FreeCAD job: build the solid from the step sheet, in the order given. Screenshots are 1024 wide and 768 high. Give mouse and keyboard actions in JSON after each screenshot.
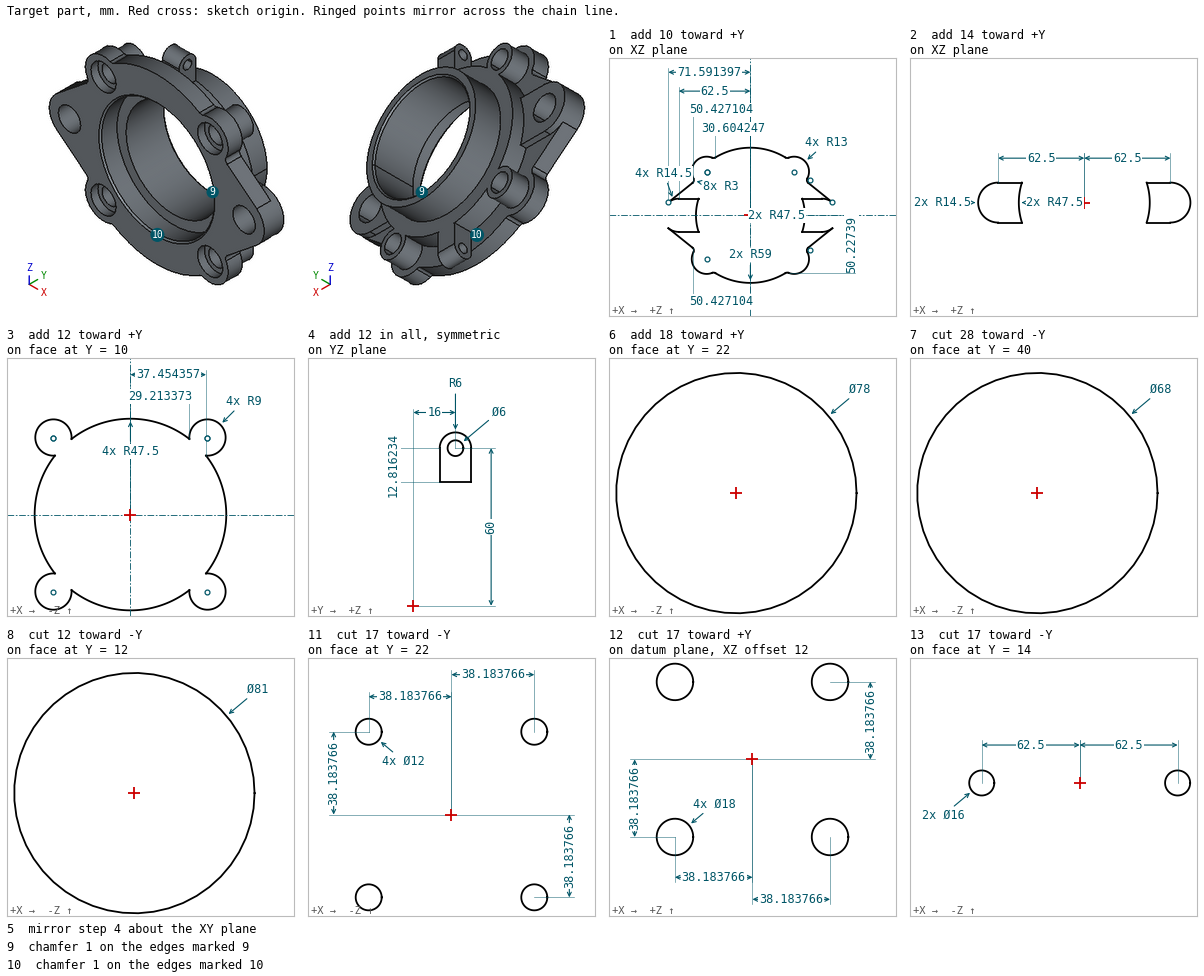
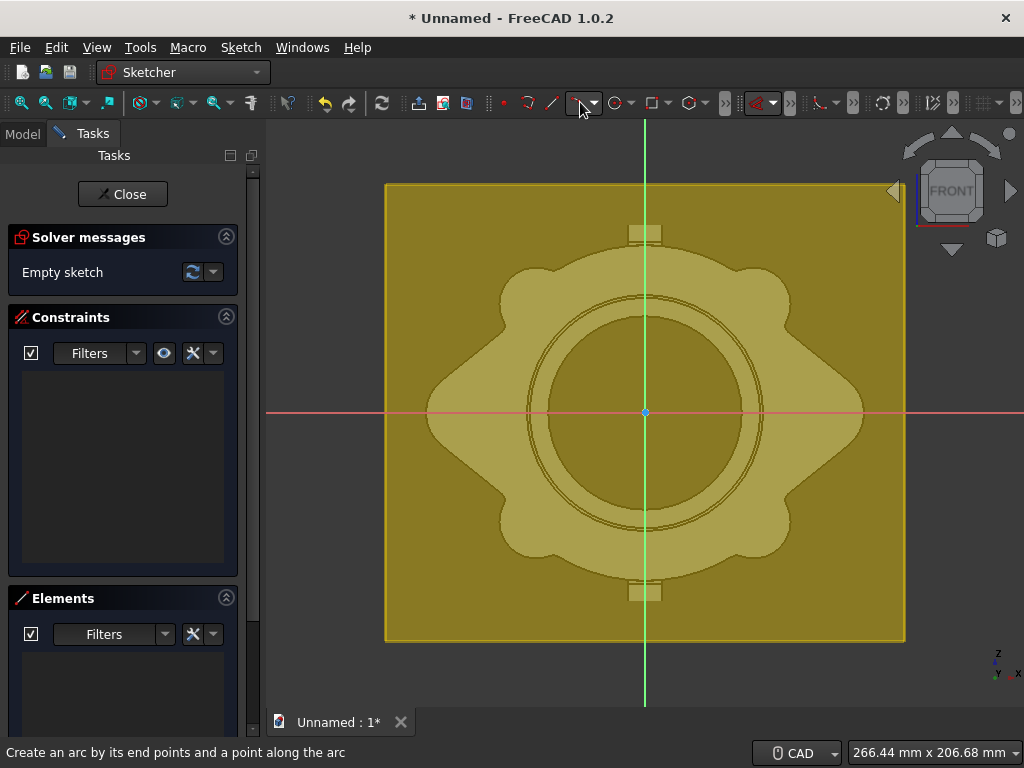
{"action": "scroll", "coordinate": [784, 413], "scroll_direction": "up", "scroll_amount": 2}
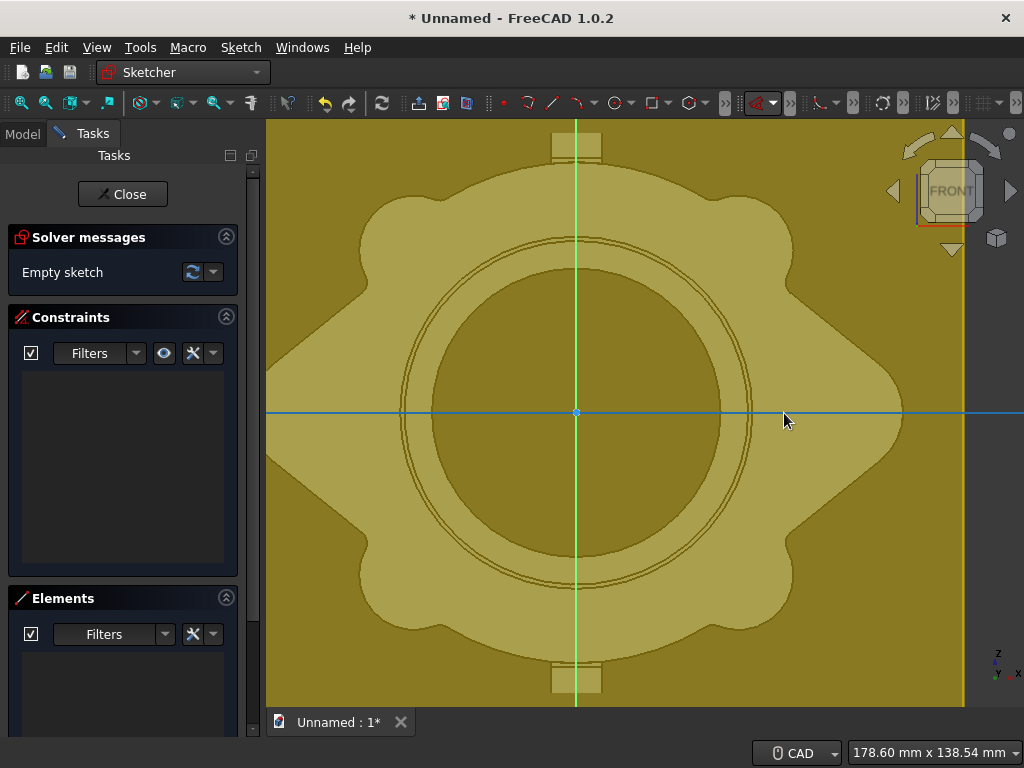
{"action": "key", "text": "g c"}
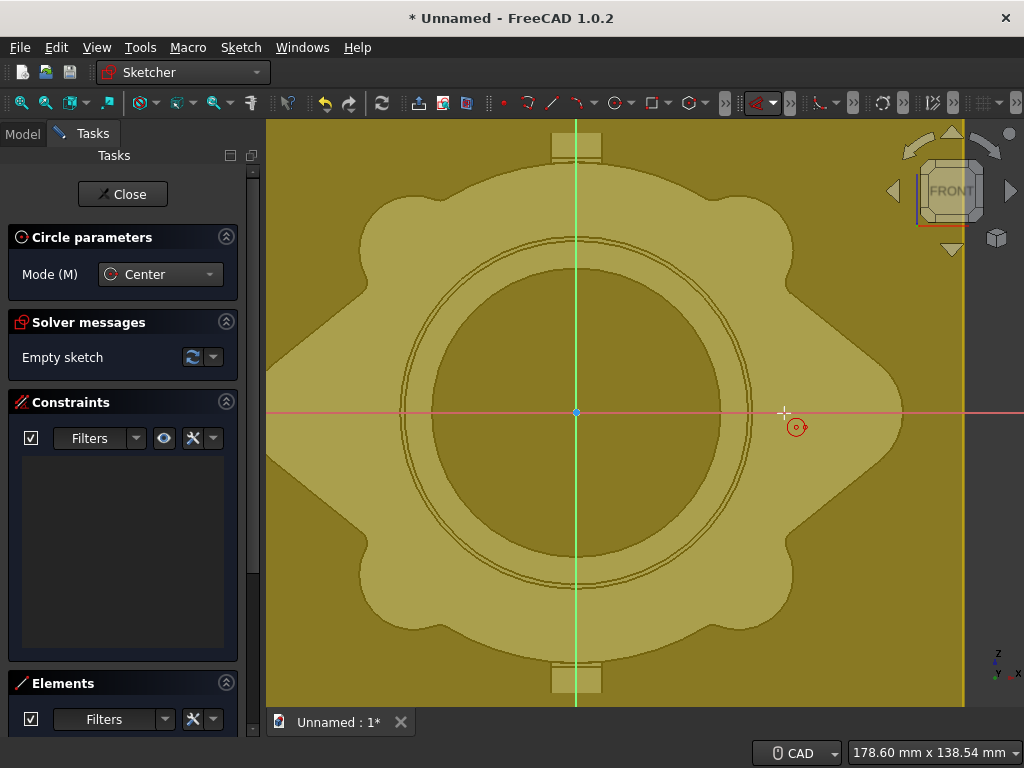
{"action": "left_click", "coordinate": [414, 575]}
{"action": "left_click", "coordinate": [441, 548]}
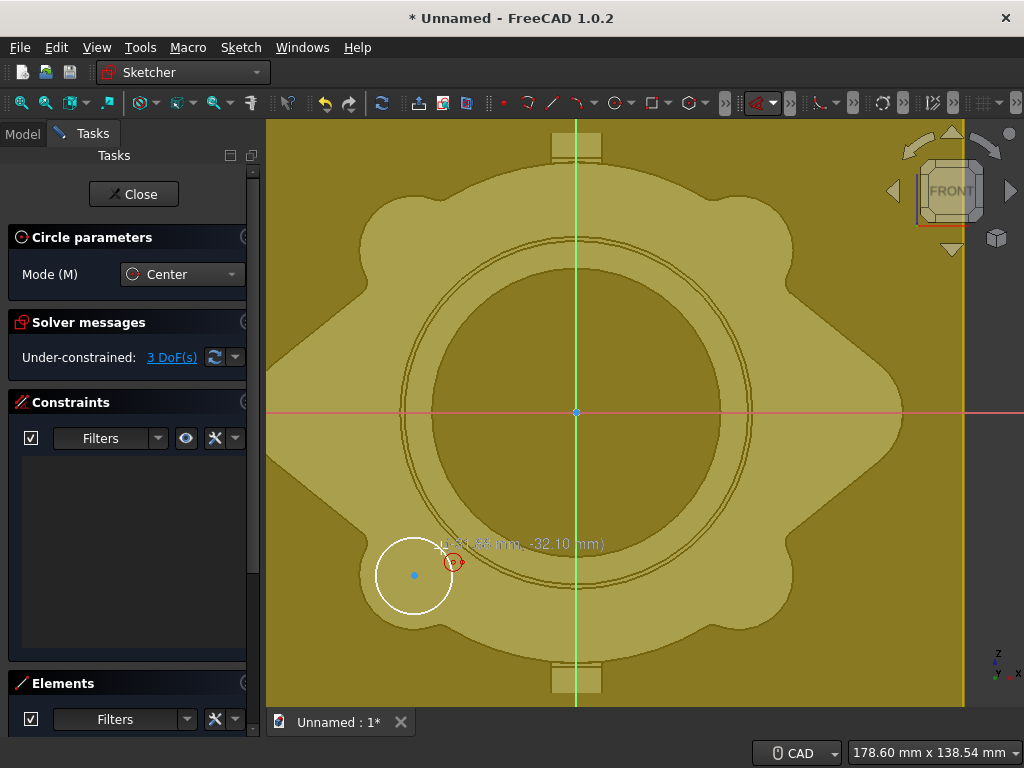
{"action": "left_click", "coordinate": [738, 575]}
{"action": "left_click", "coordinate": [765, 548]}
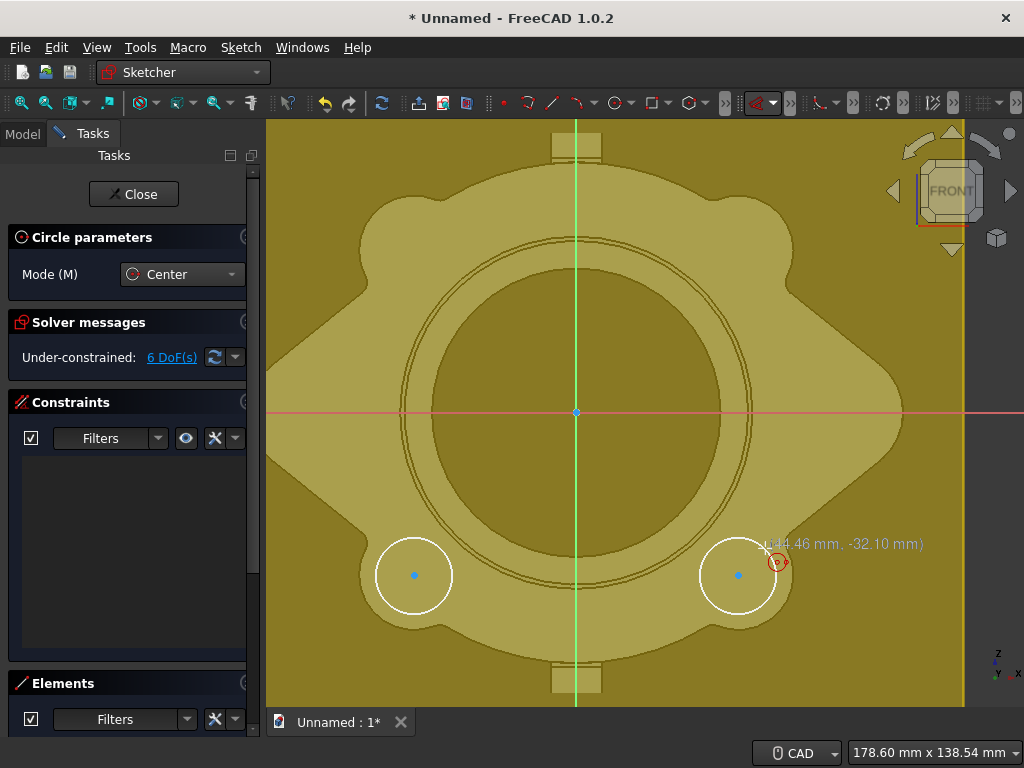
{"action": "left_click", "coordinate": [738, 251]}
{"action": "left_click", "coordinate": [765, 224]}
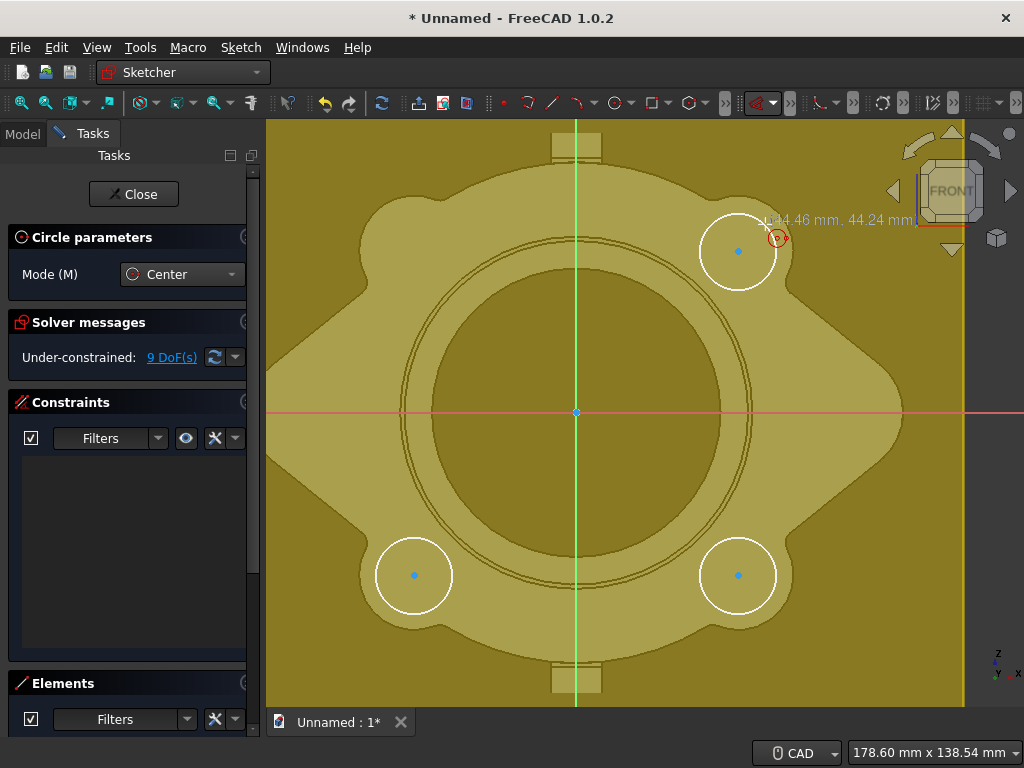
{"action": "left_click", "coordinate": [414, 251]}
{"action": "left_click", "coordinate": [441, 224]}
{"action": "key", "text": "Escape"}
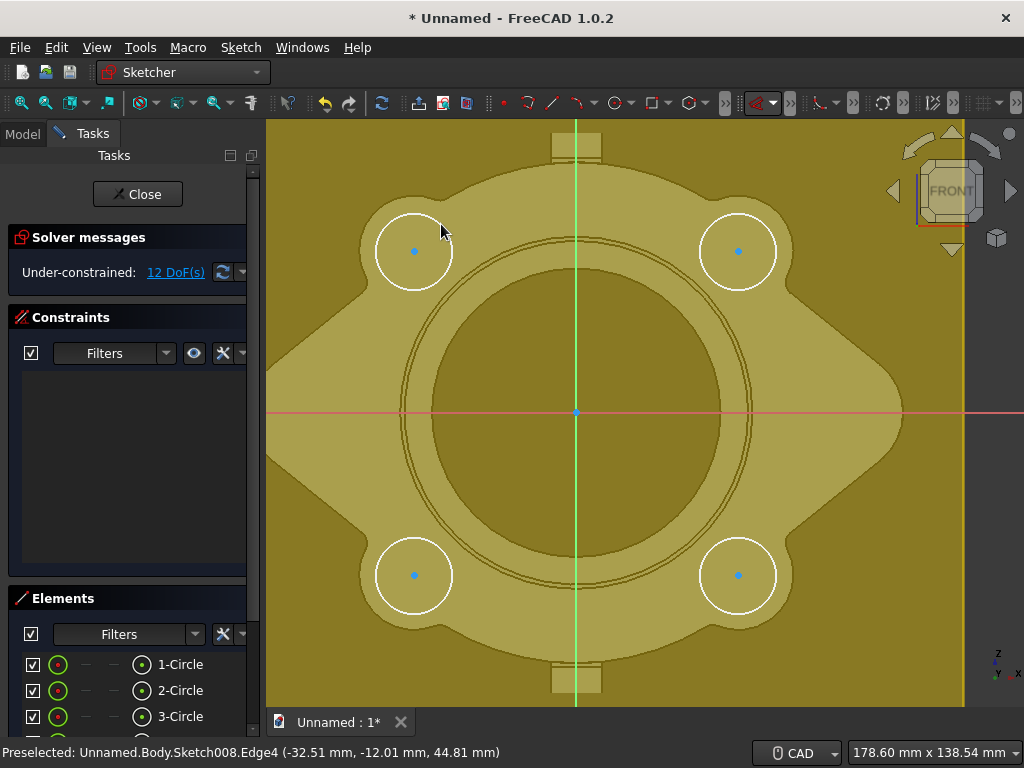
{"action": "left_click", "coordinate": [441, 549]}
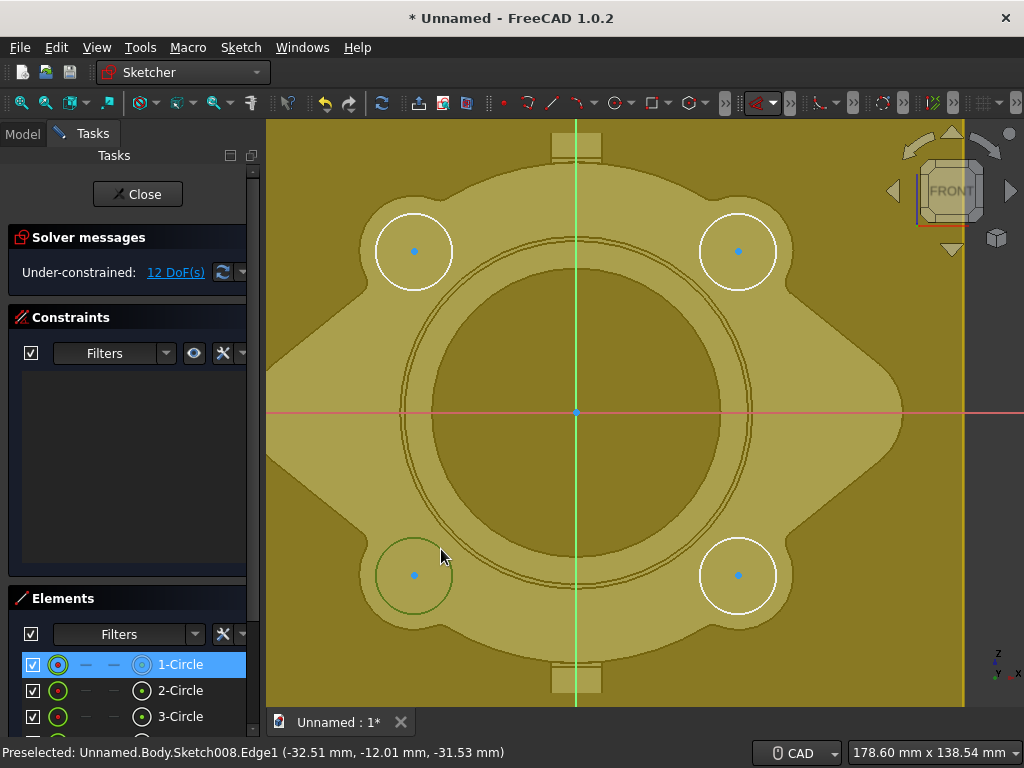
{"action": "left_click", "coordinate": [765, 549]}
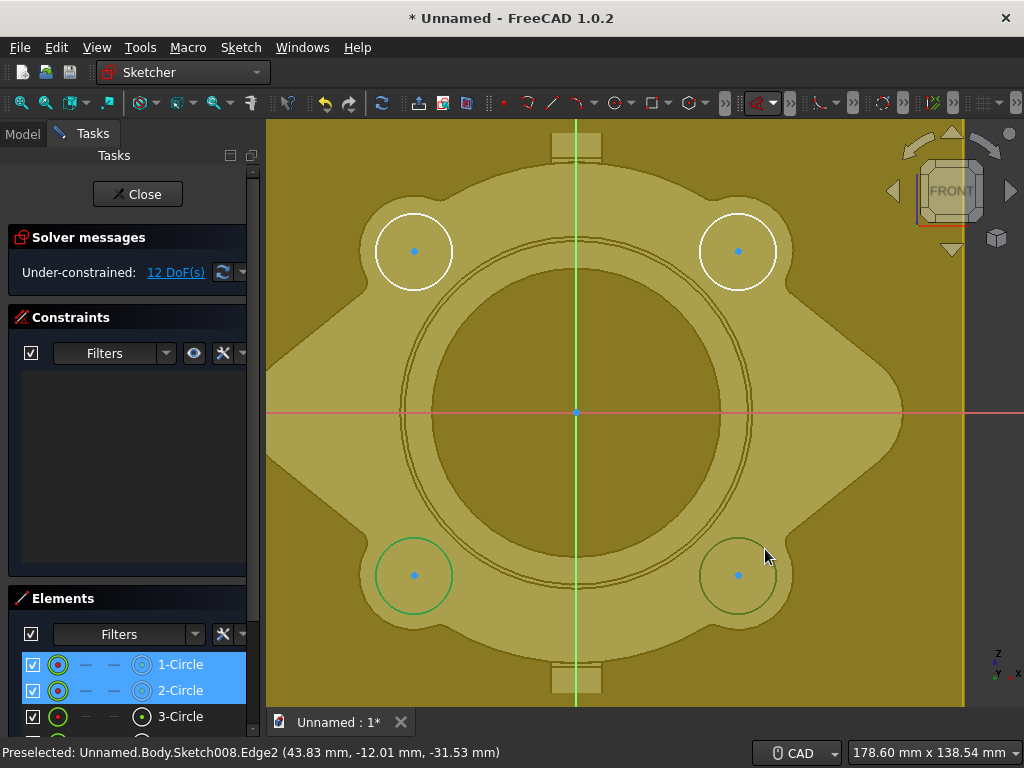
{"action": "left_click", "coordinate": [765, 225]}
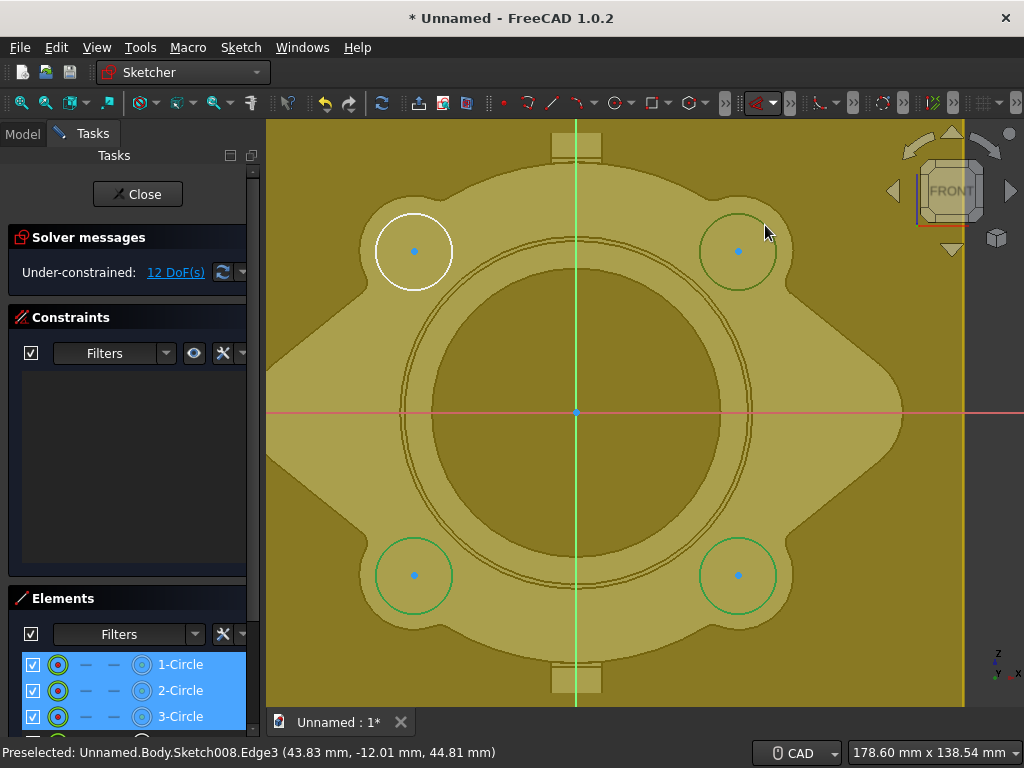
{"action": "left_click", "coordinate": [441, 225]}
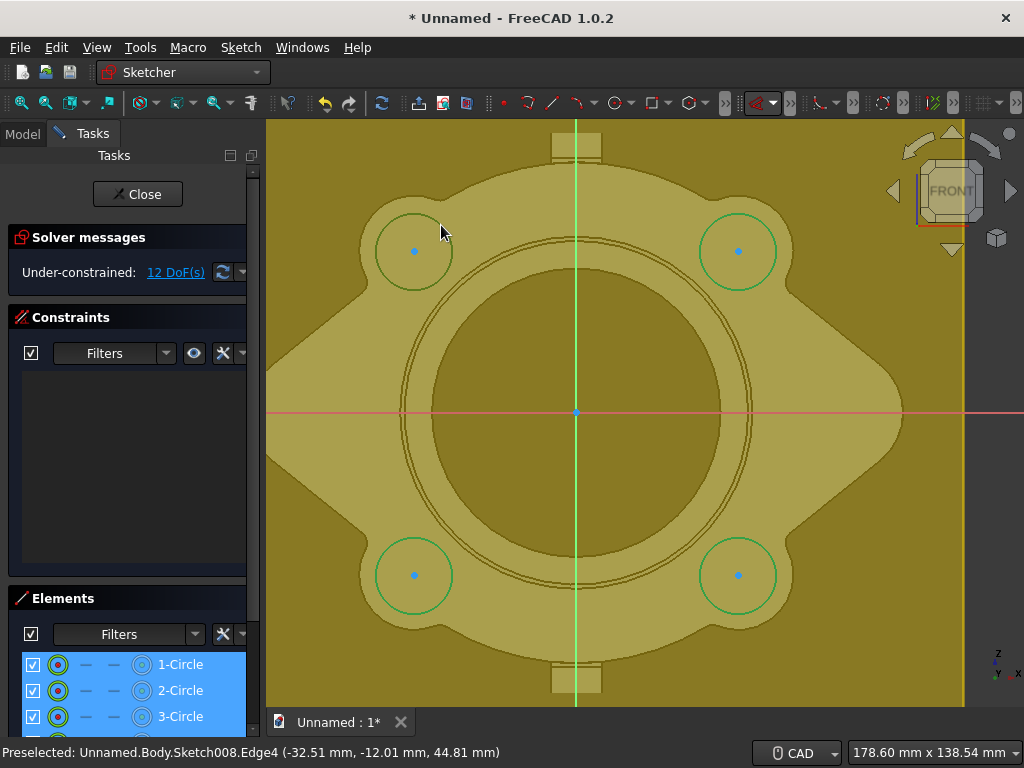
{"action": "key", "text": "e"}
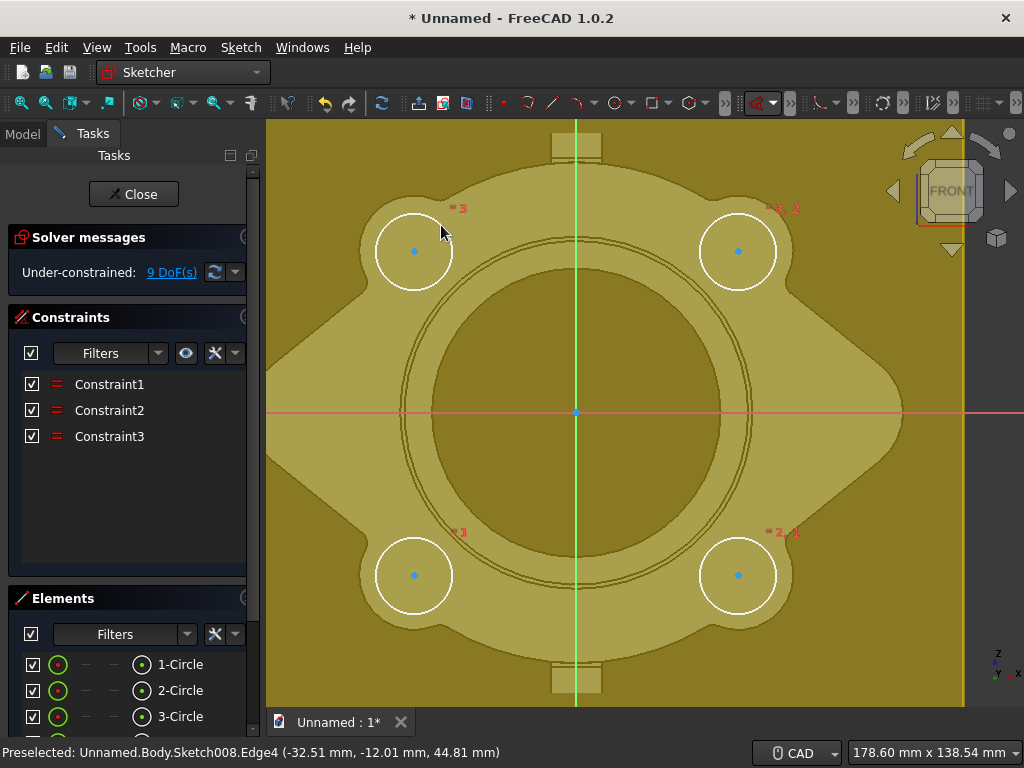
{"action": "left_click", "coordinate": [414, 576]}